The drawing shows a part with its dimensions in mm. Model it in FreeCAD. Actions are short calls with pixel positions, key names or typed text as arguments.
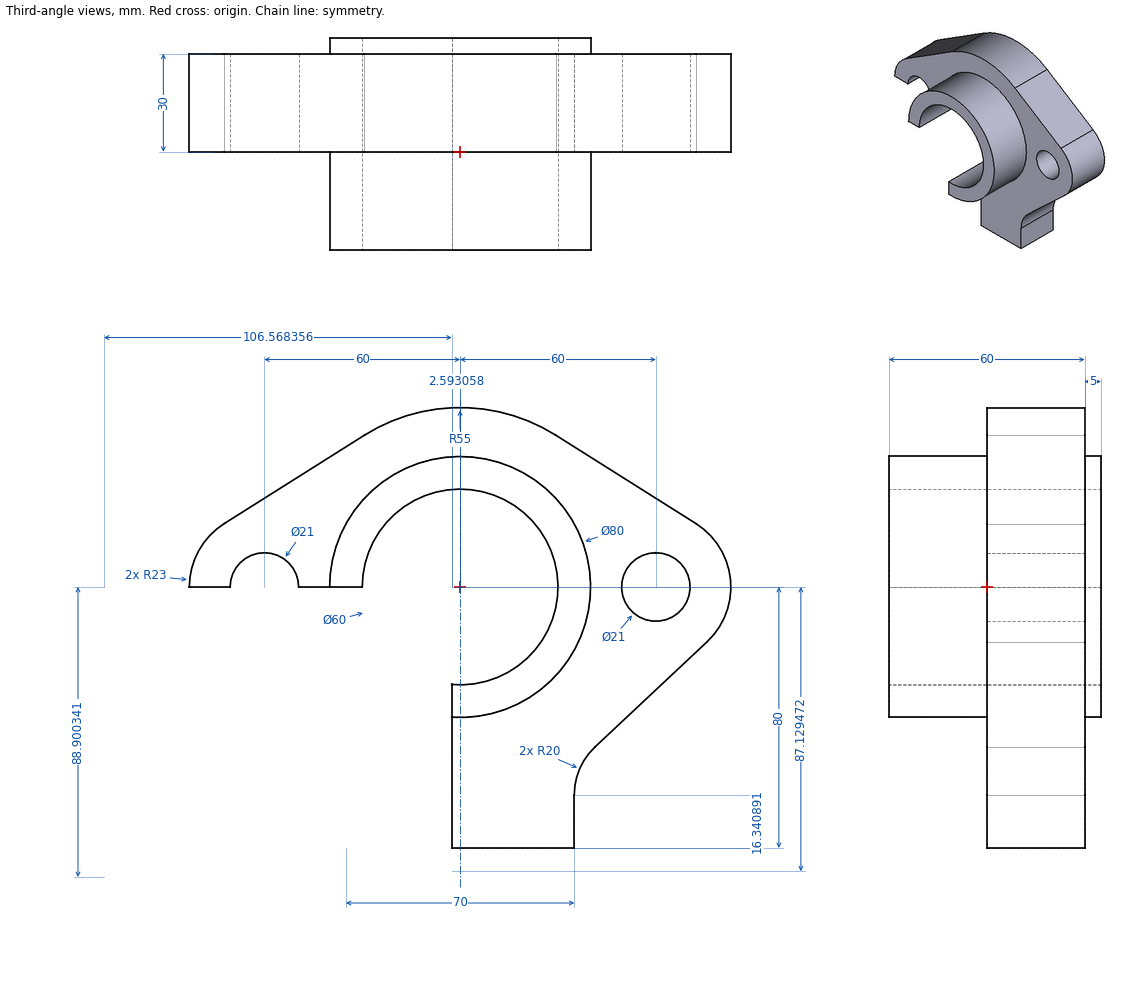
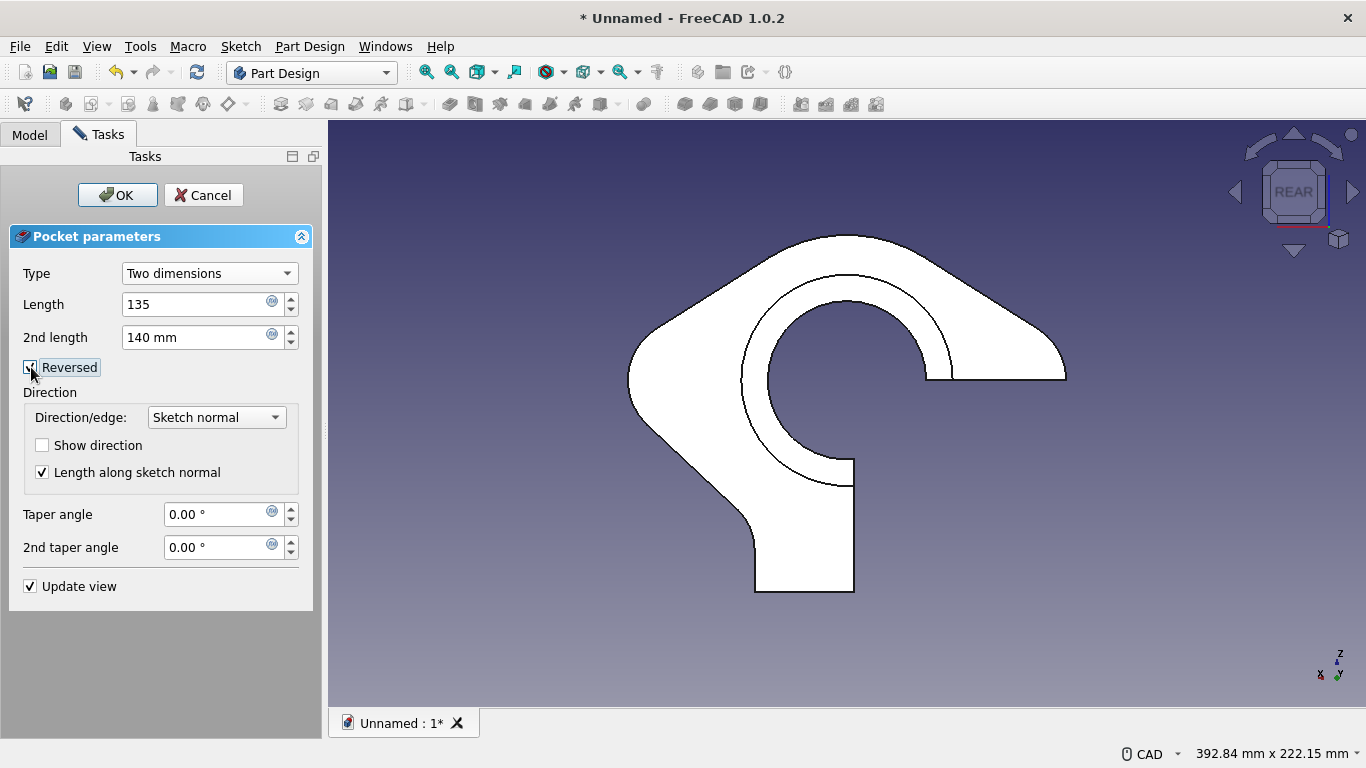
click(118, 195)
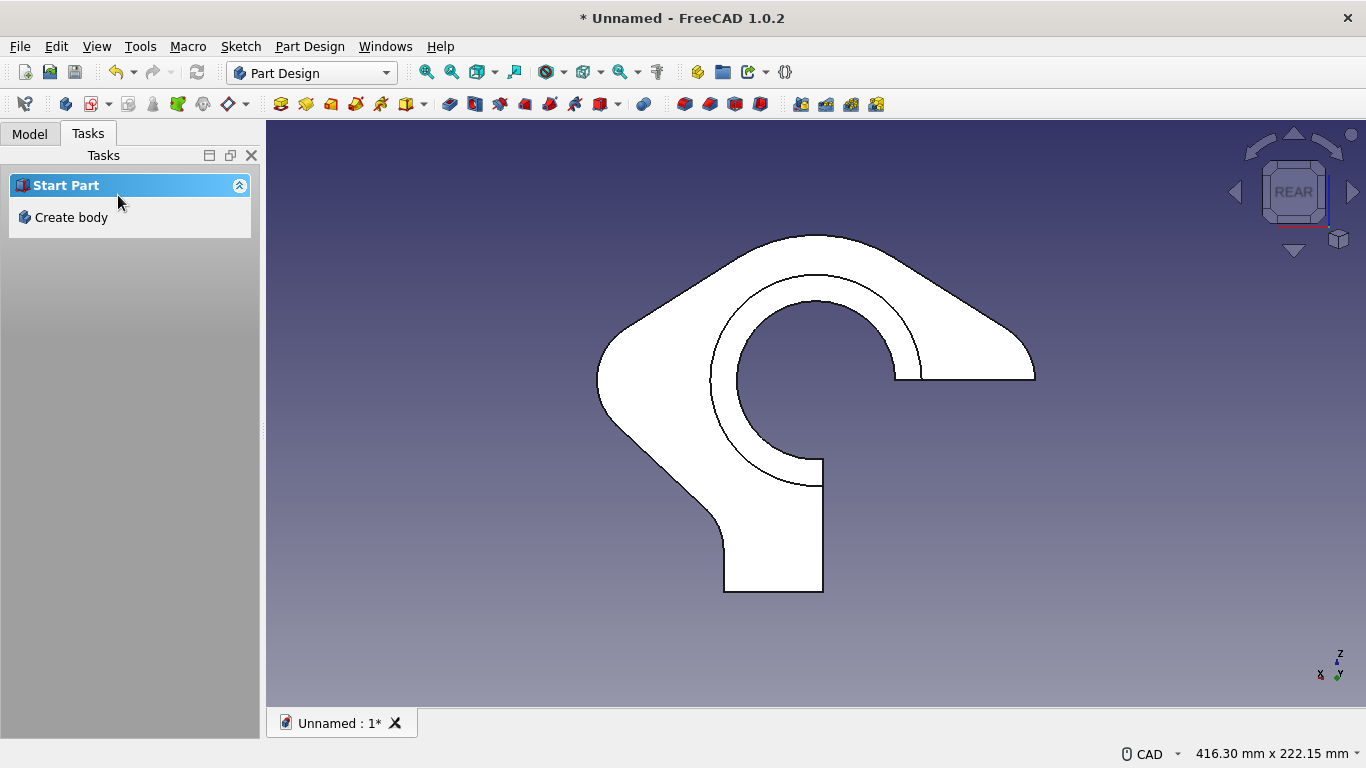
click(90, 104)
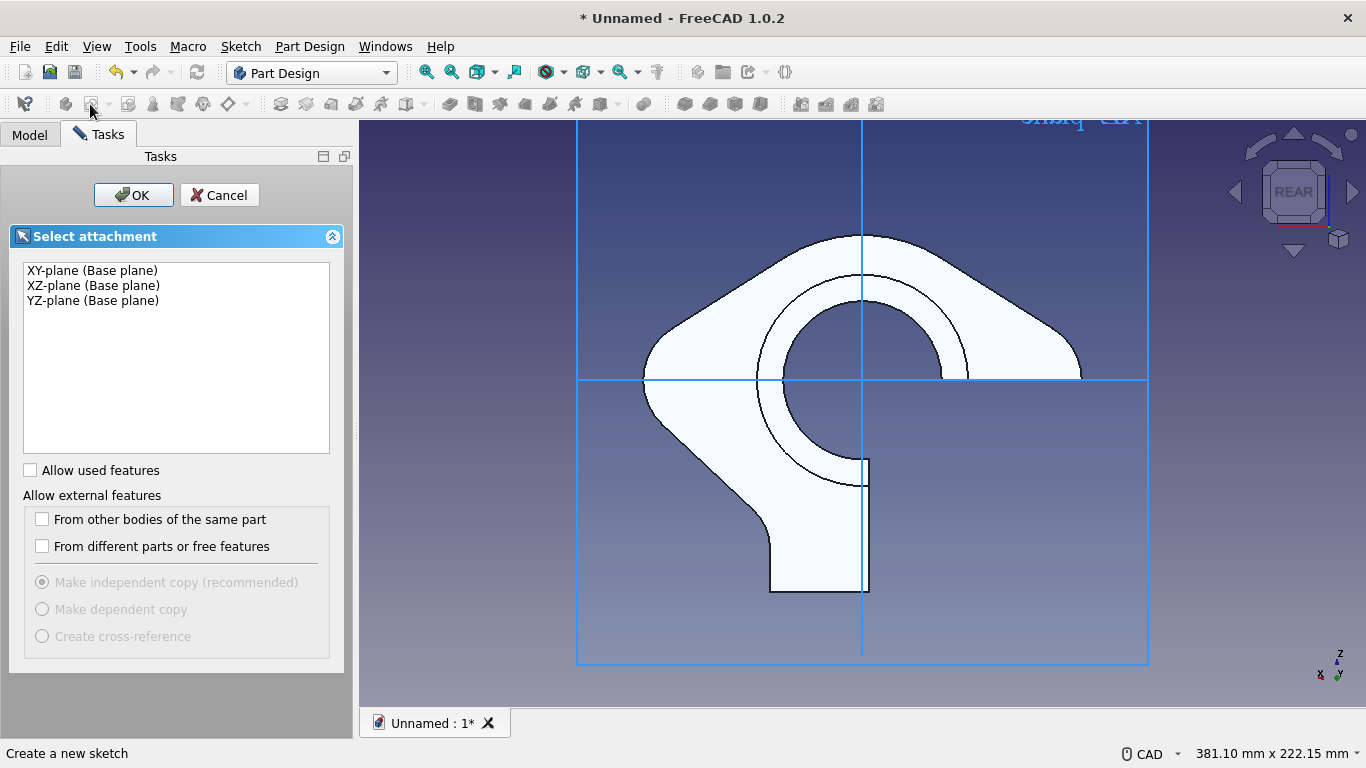
click(84, 286)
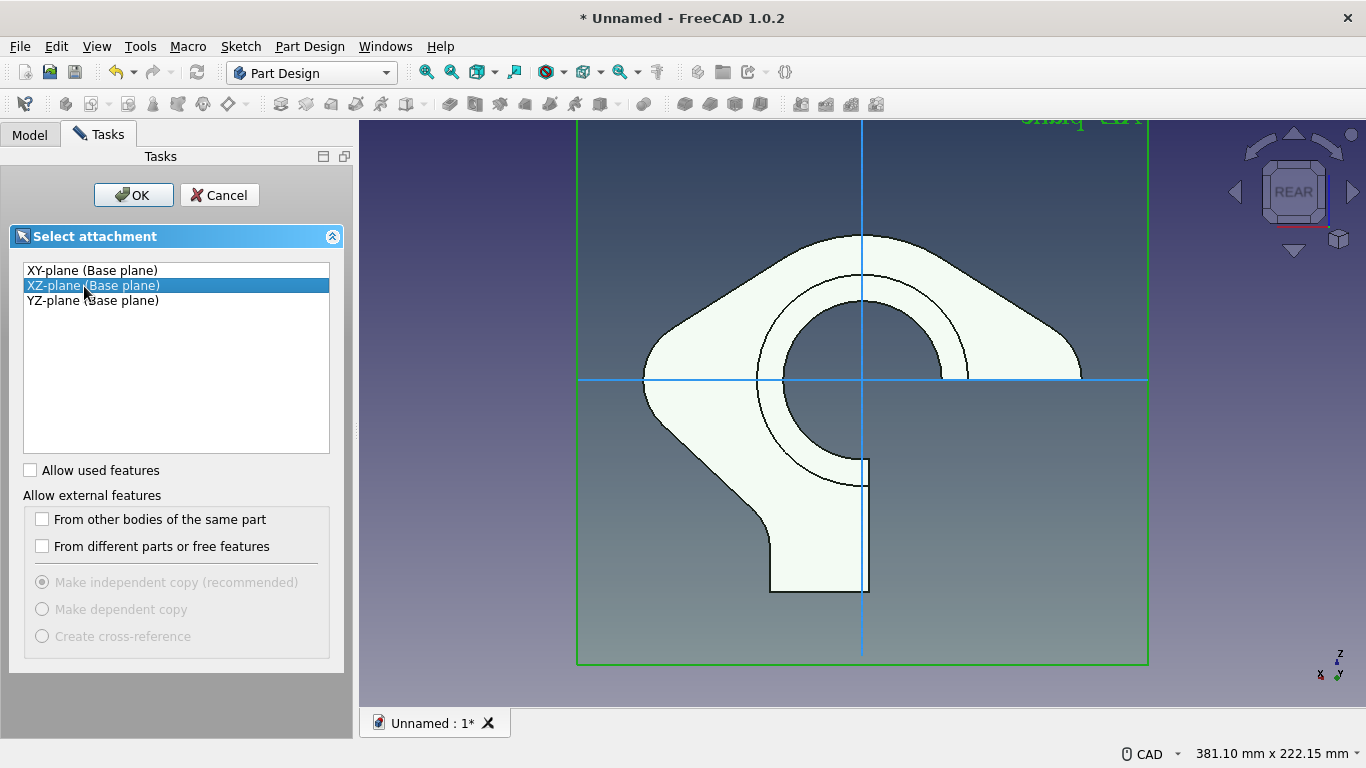
click(134, 195)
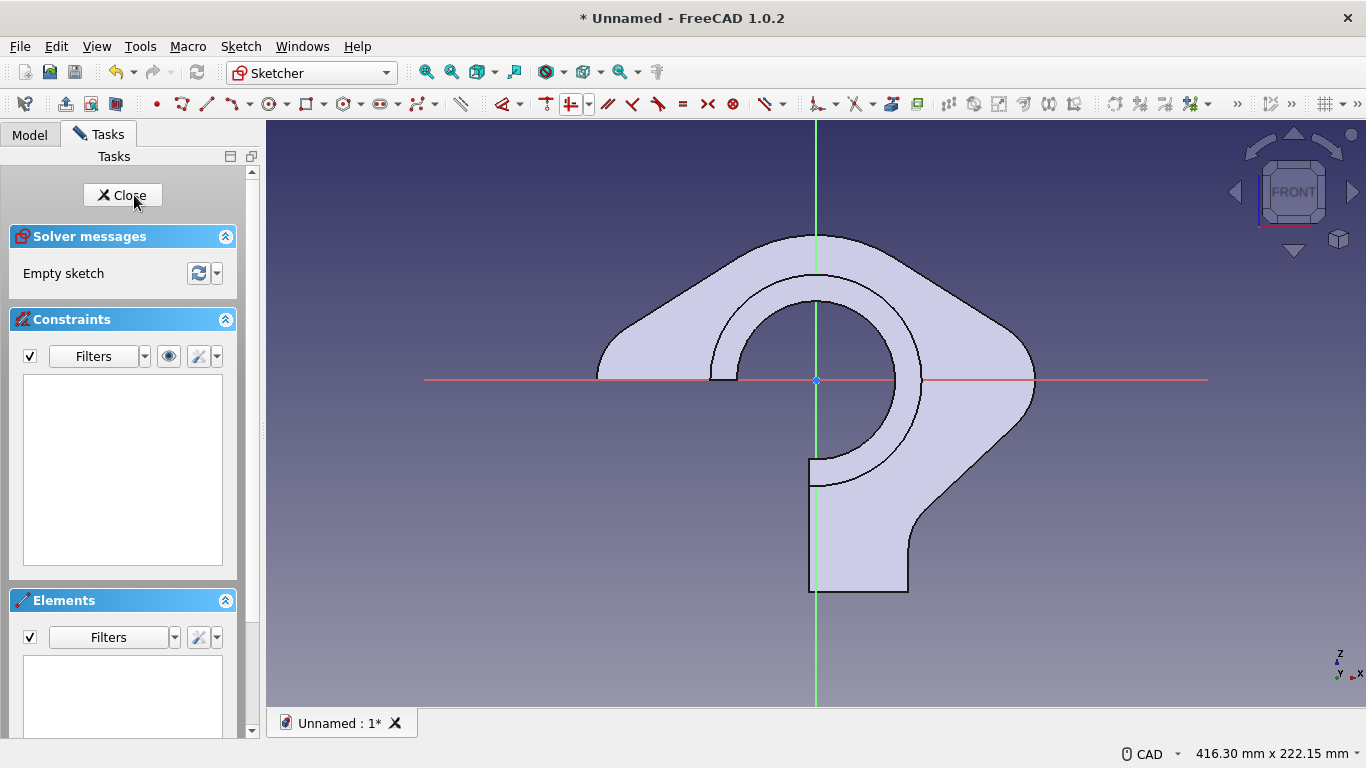
click(116, 104)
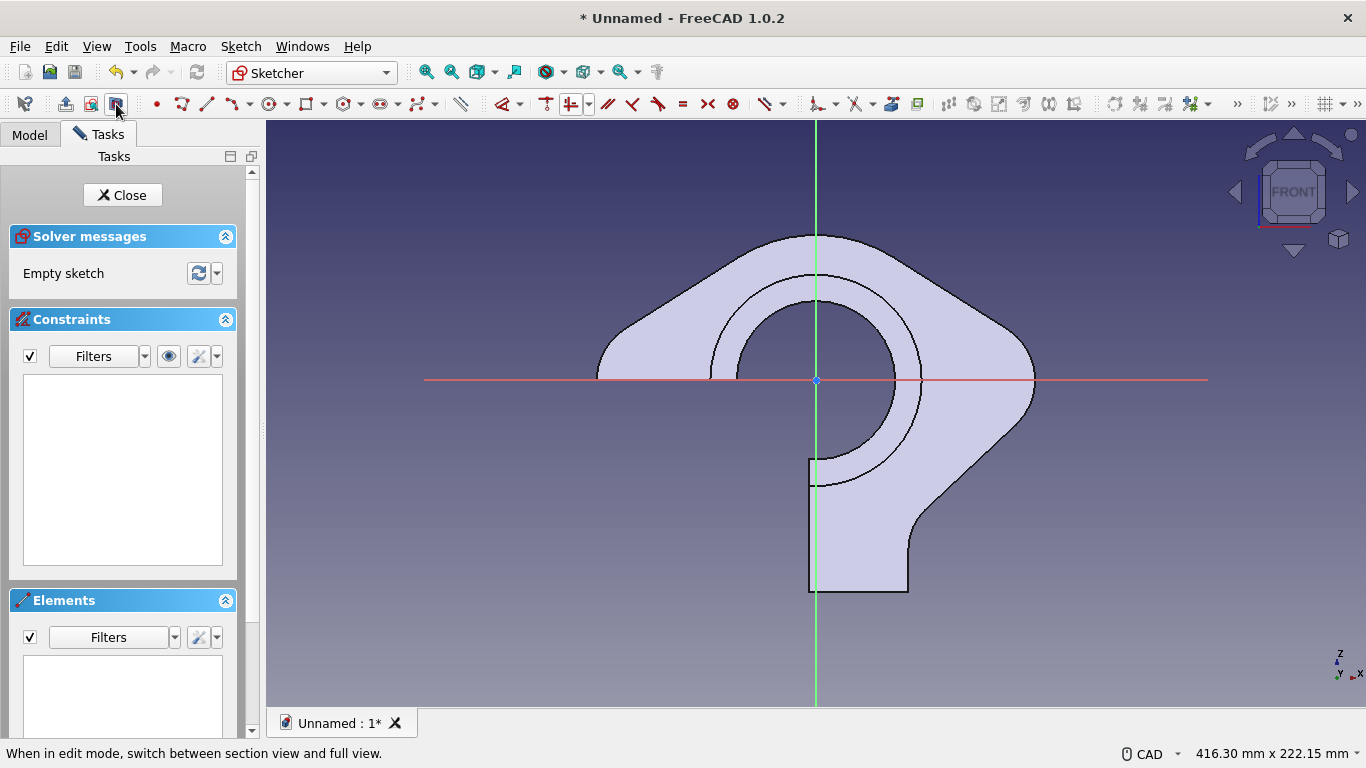
scroll(1010, 375, up, 10)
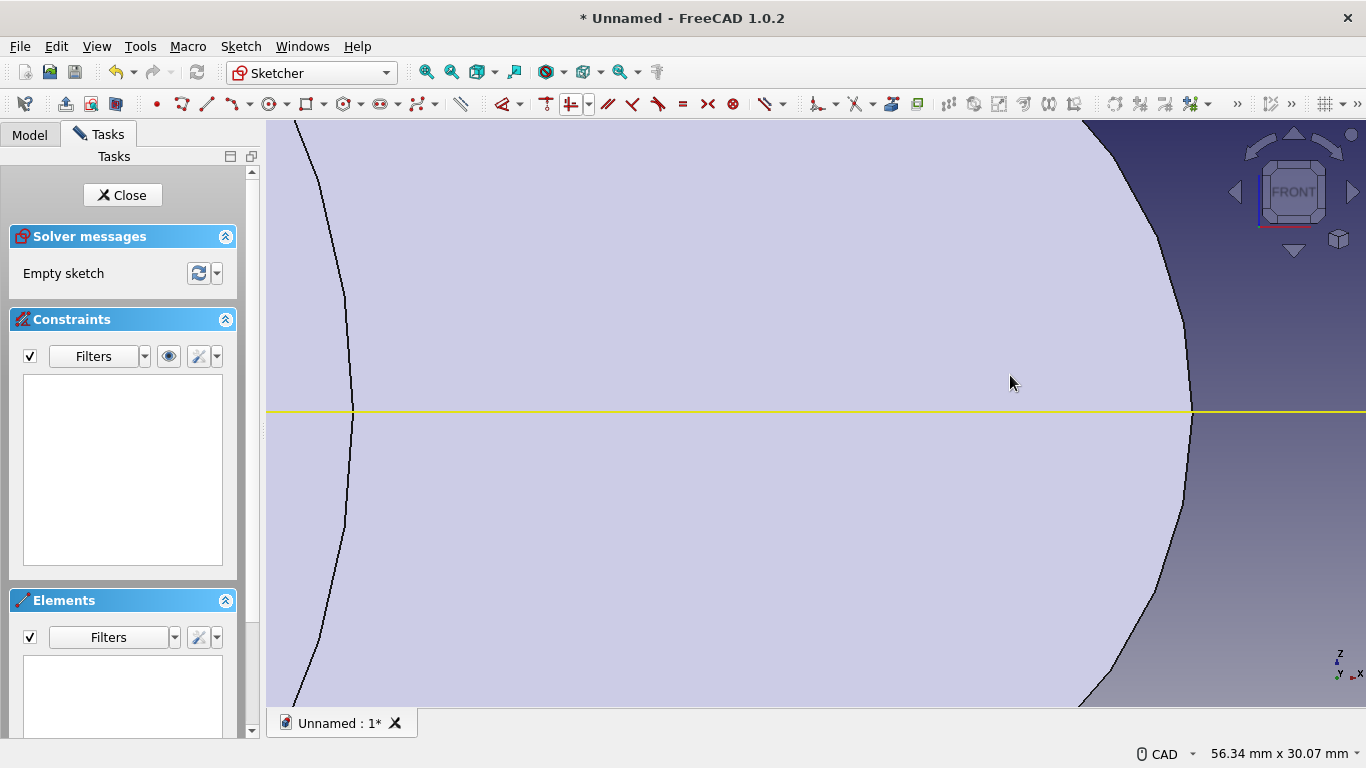
click(268, 104)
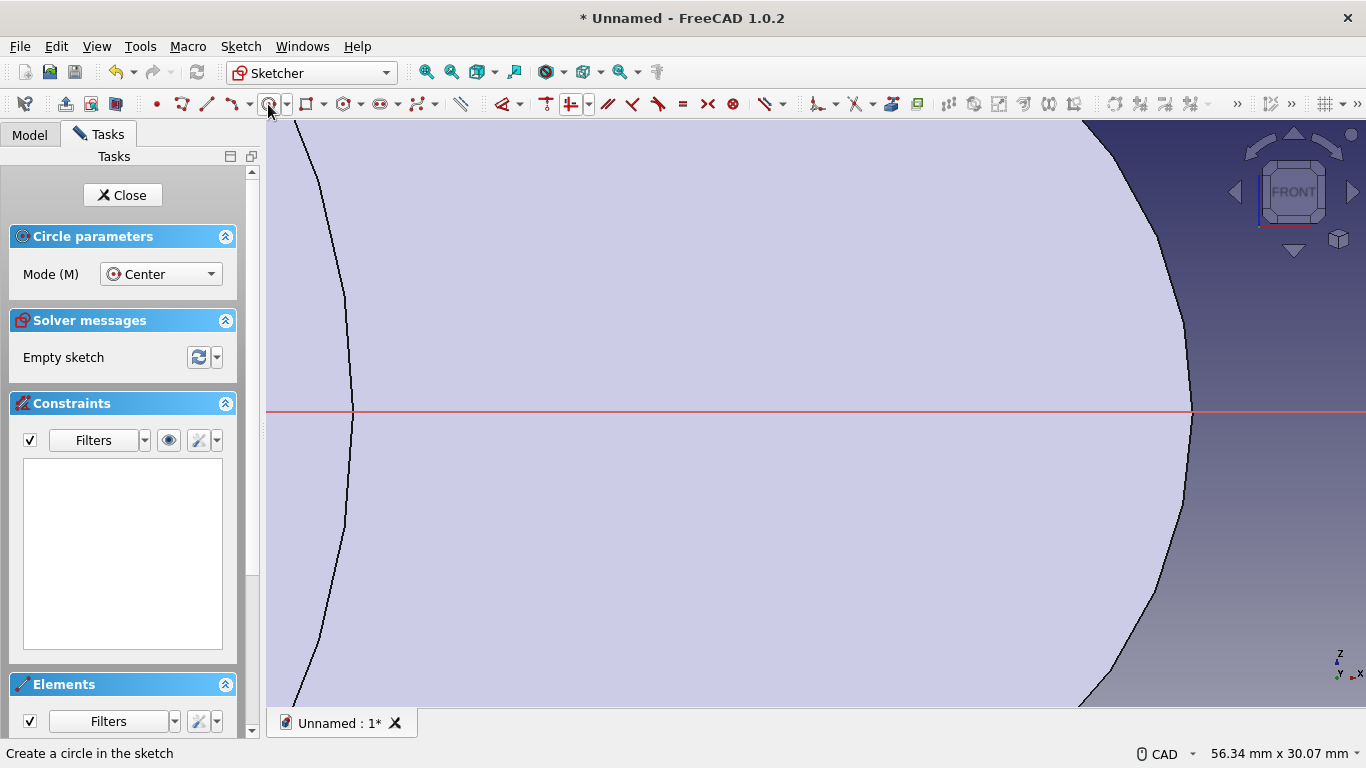
click(744, 412)
move(889, 267)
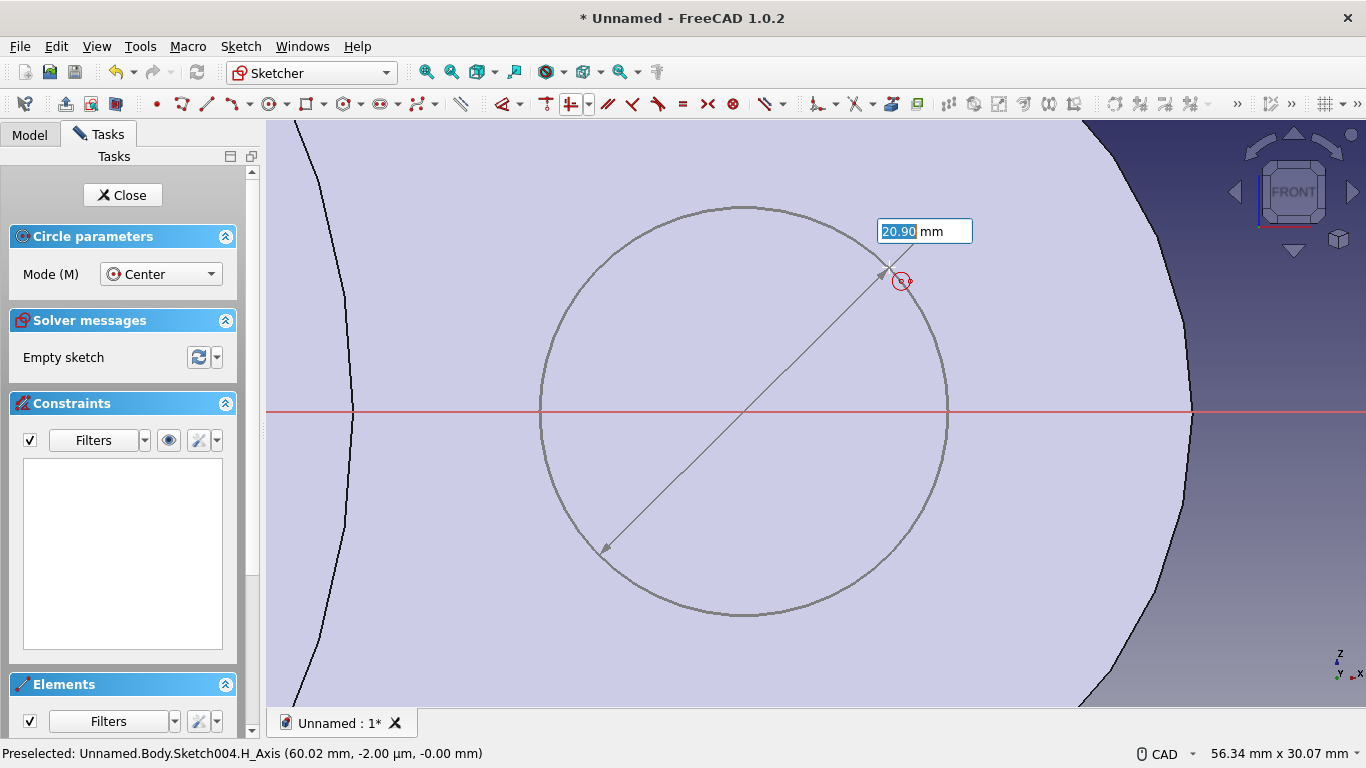
text(21)
key(Return)
key(Escape)